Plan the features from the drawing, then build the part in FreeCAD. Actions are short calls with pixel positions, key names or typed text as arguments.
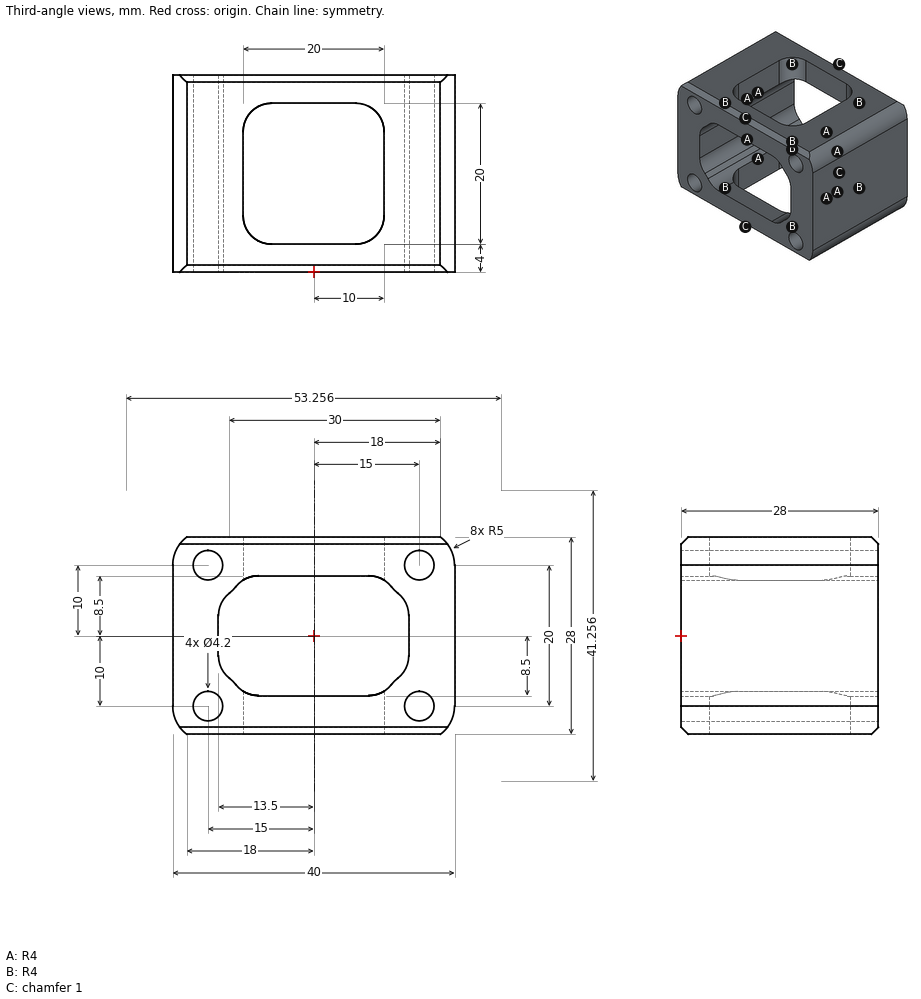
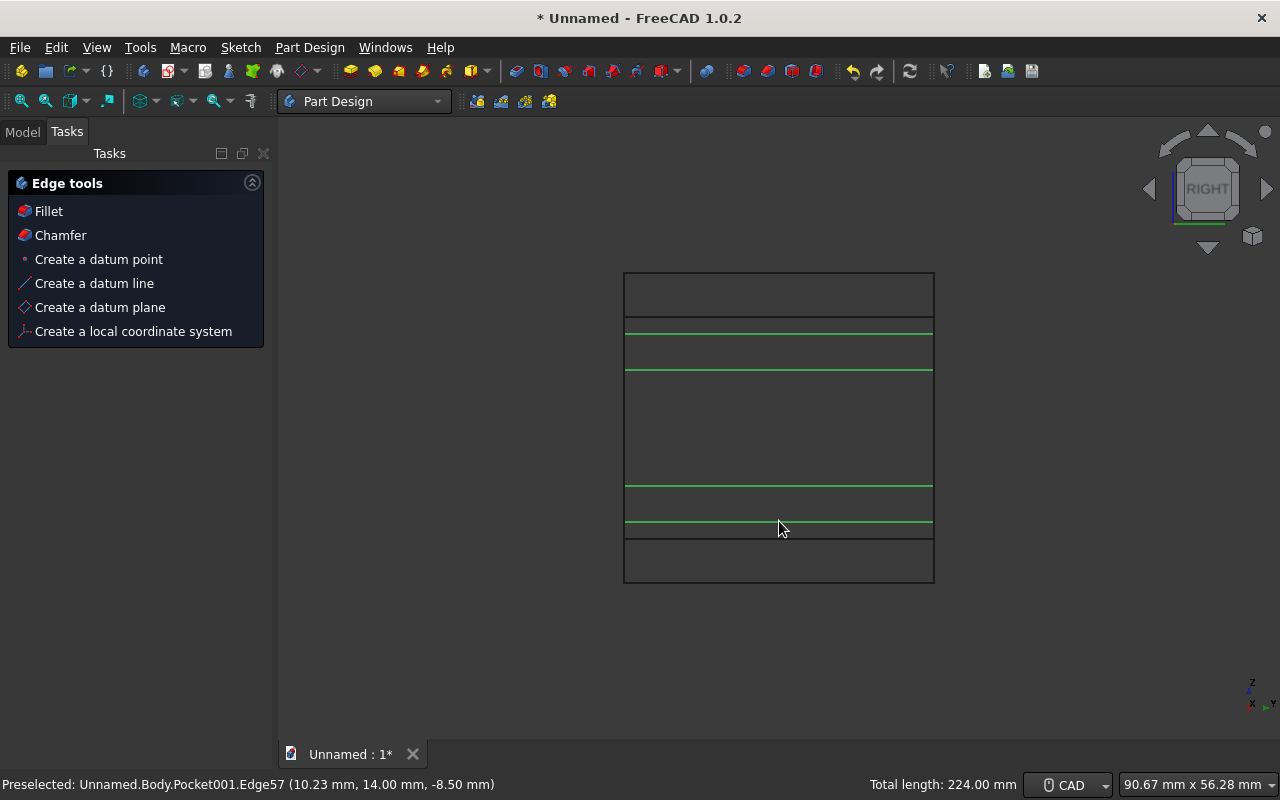
key(v)
key(1)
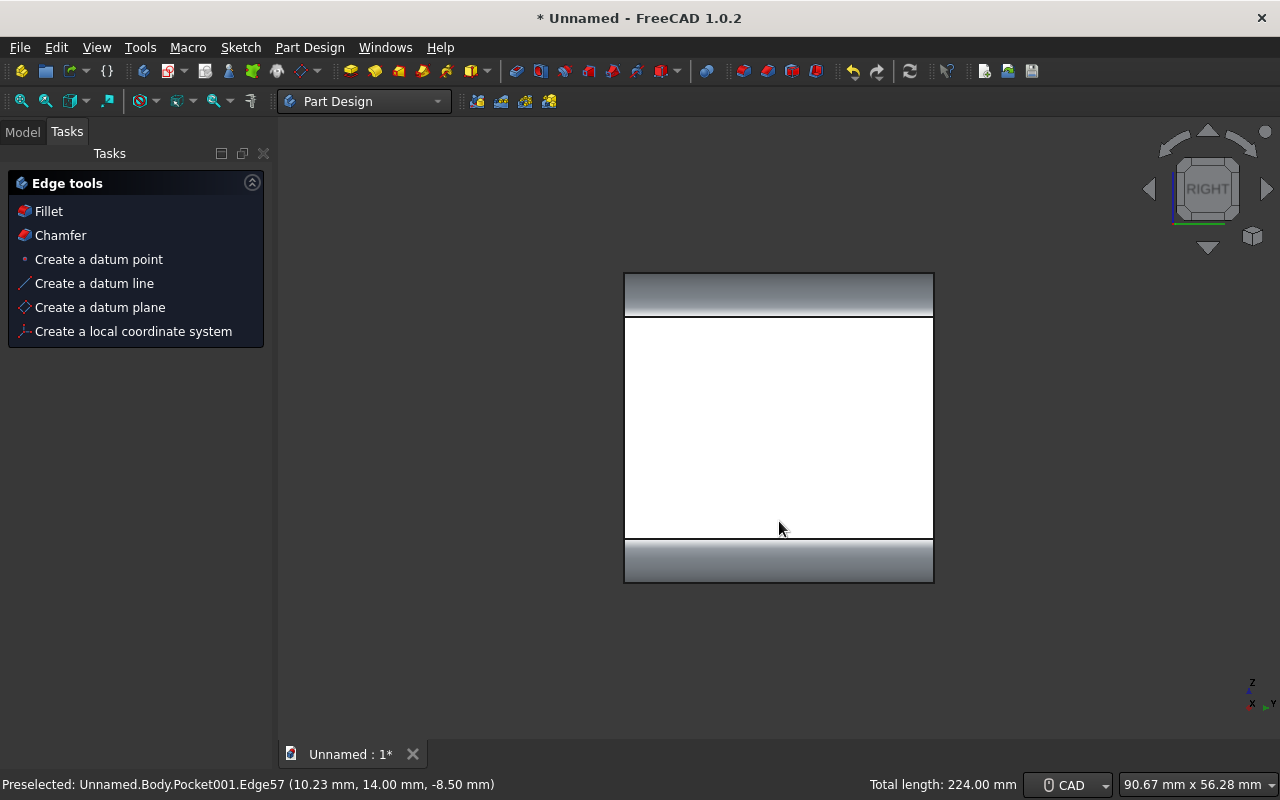
click(744, 72)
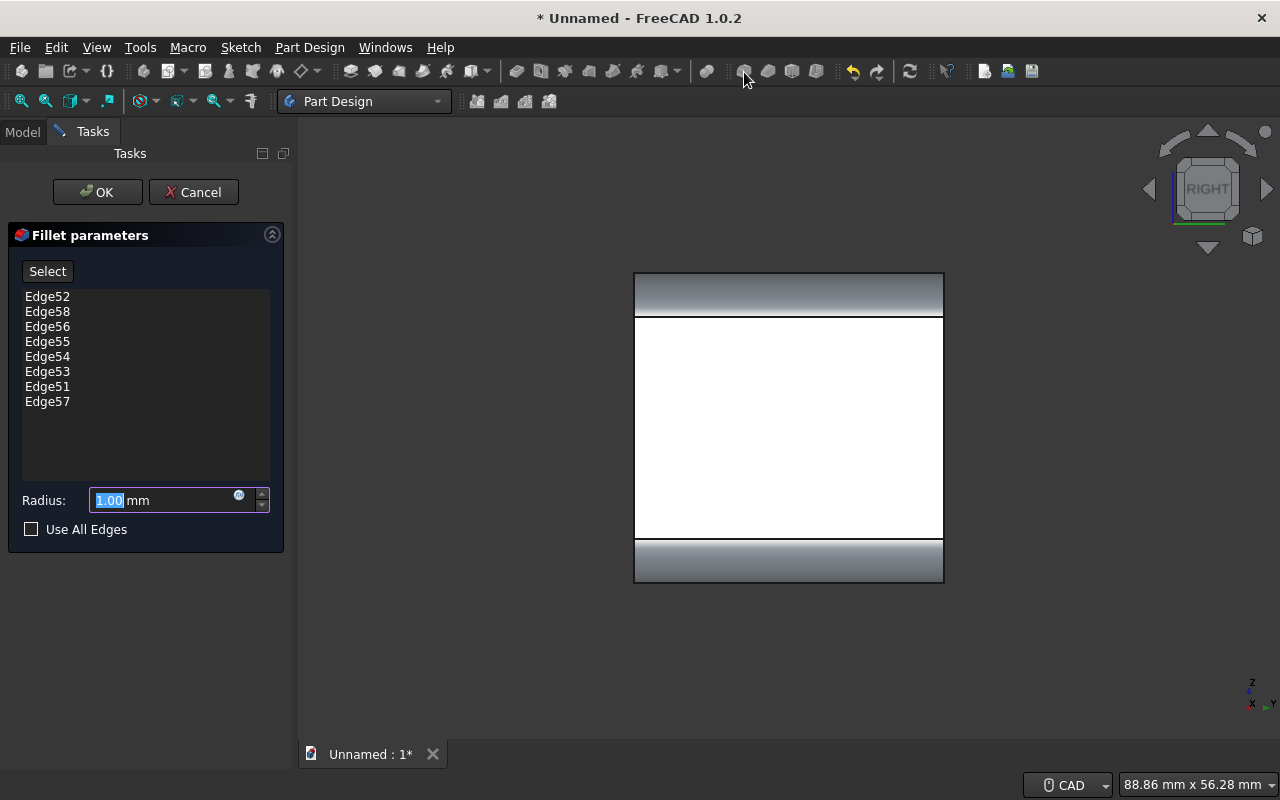
text(4)
key(Tab)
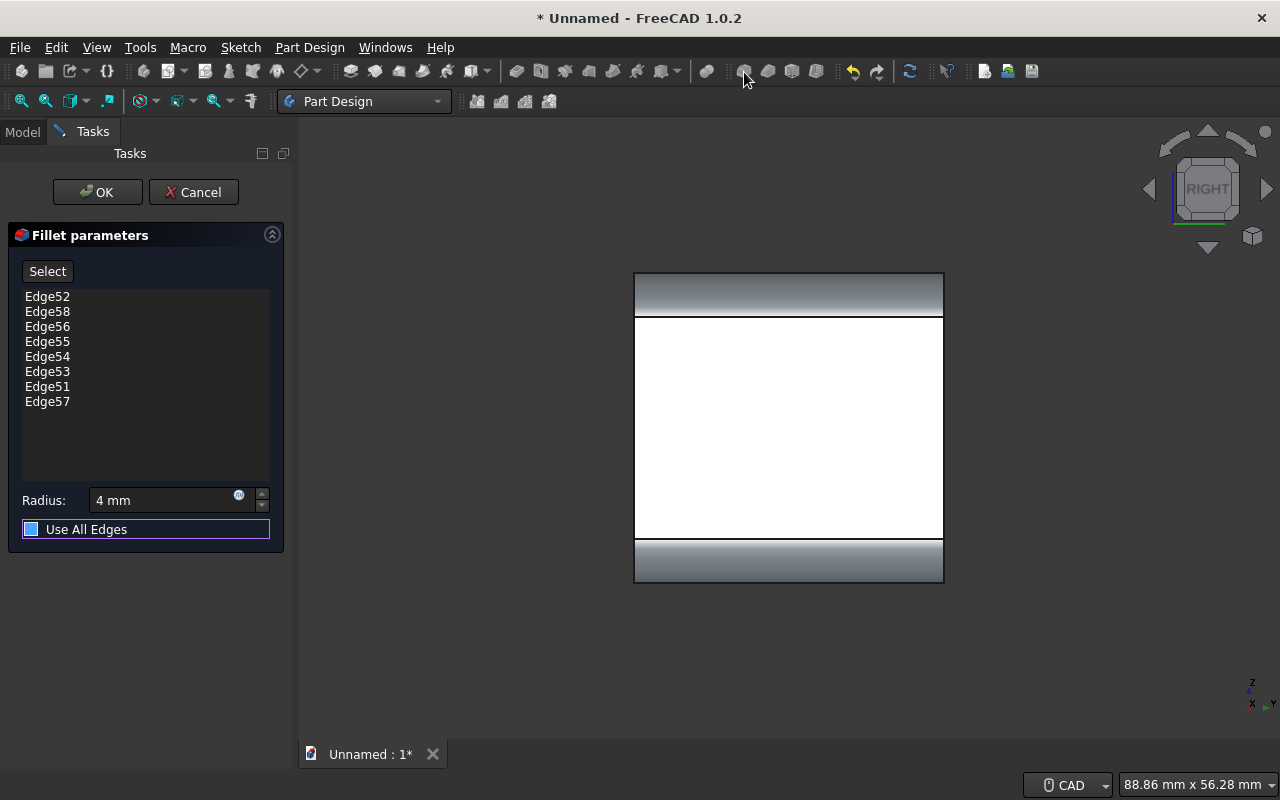
click(98, 192)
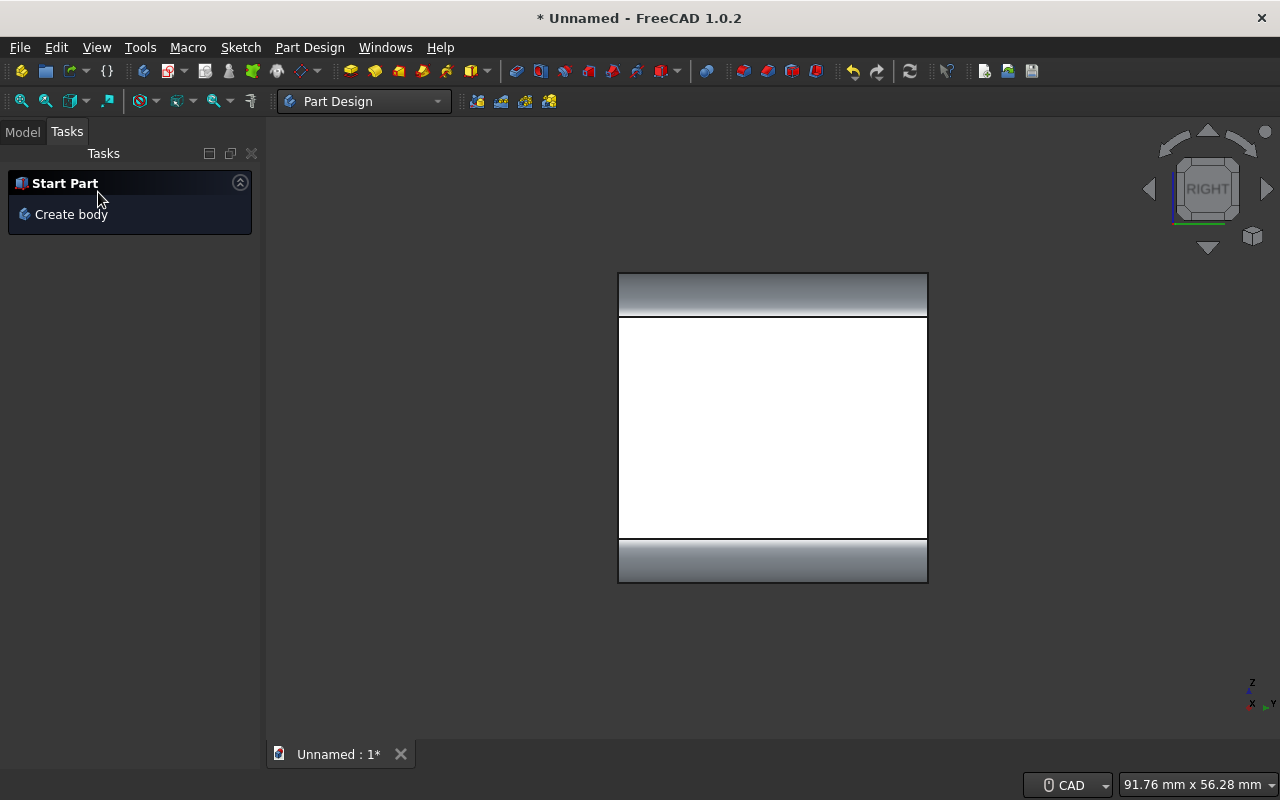
key(0)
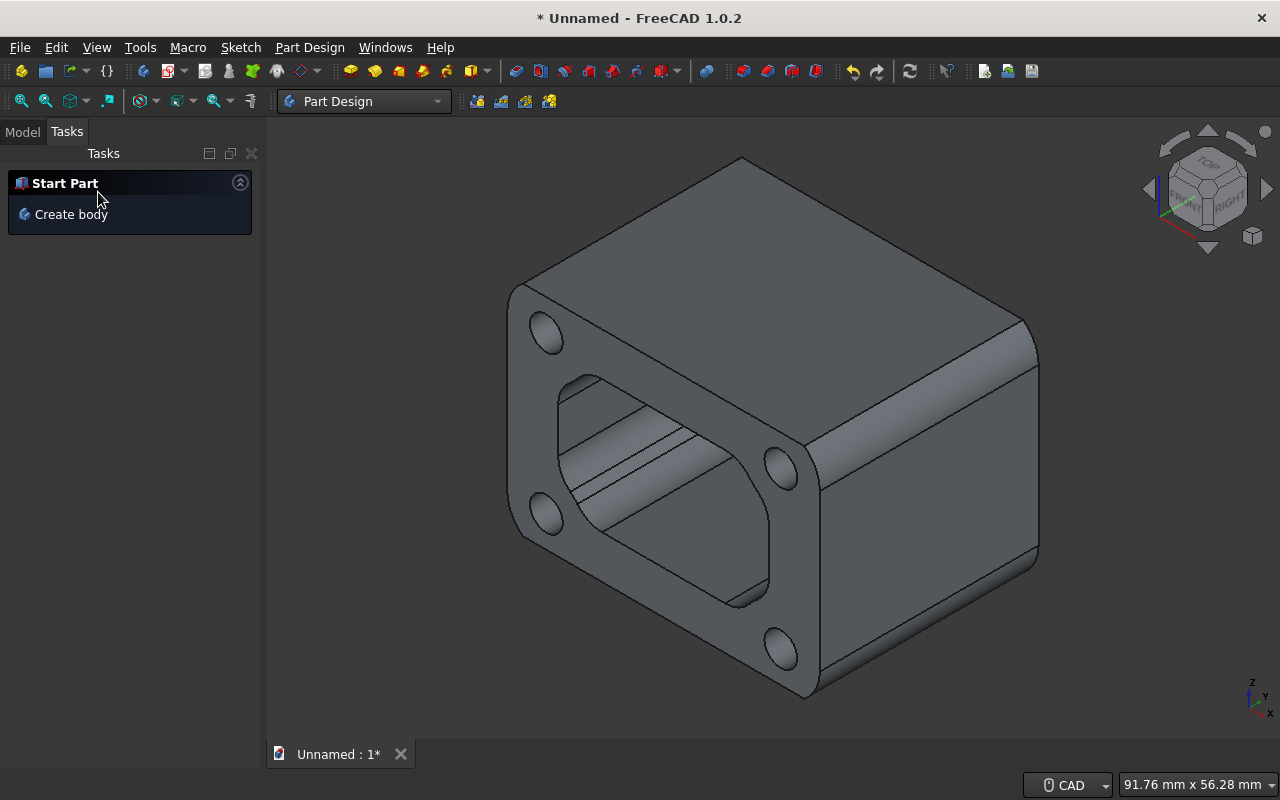
click(773, 301)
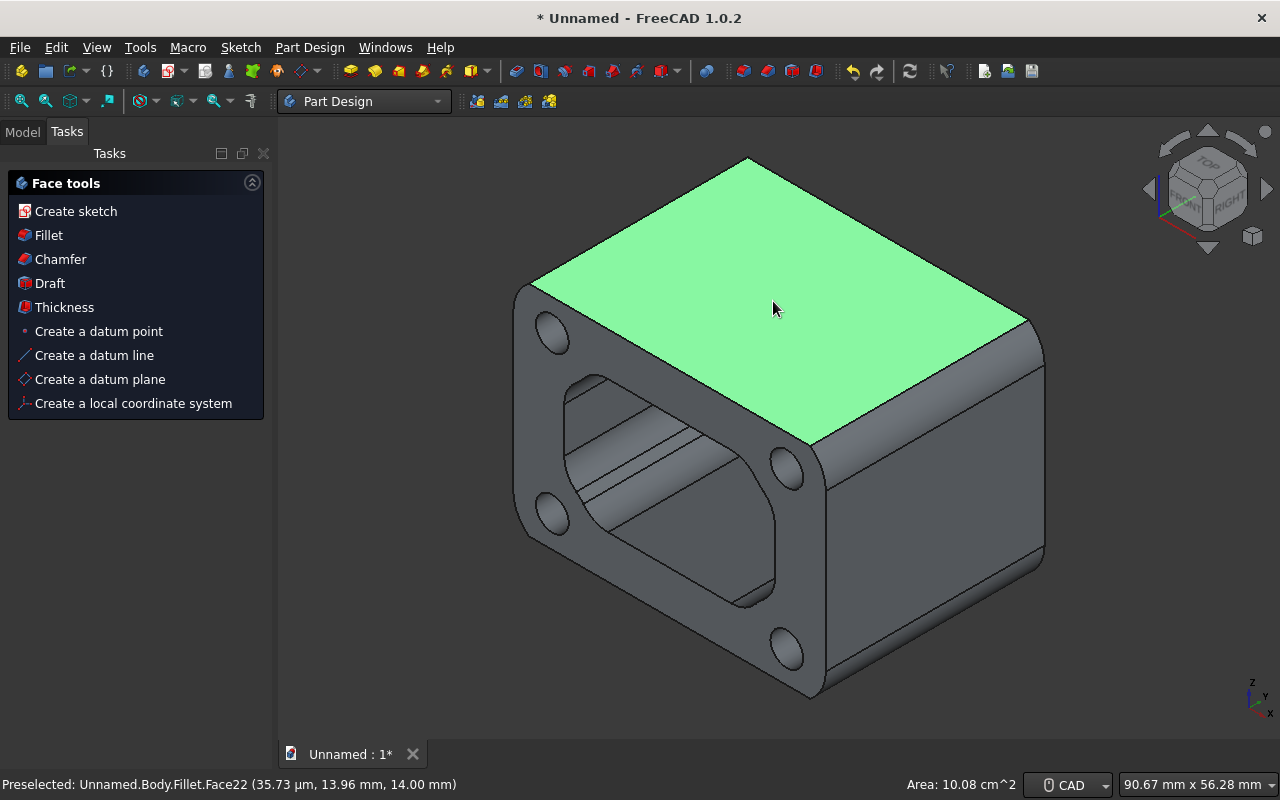
click(168, 72)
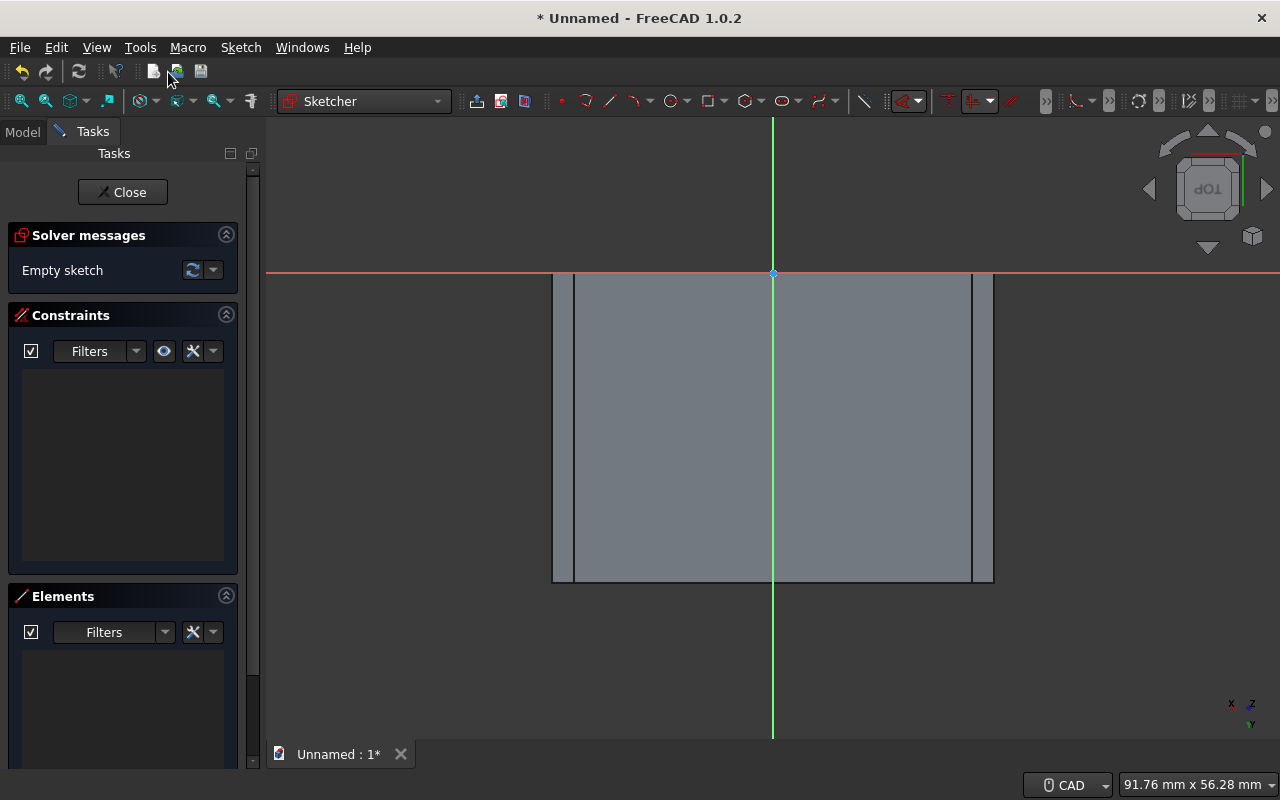
scroll(912, 361, up, 2)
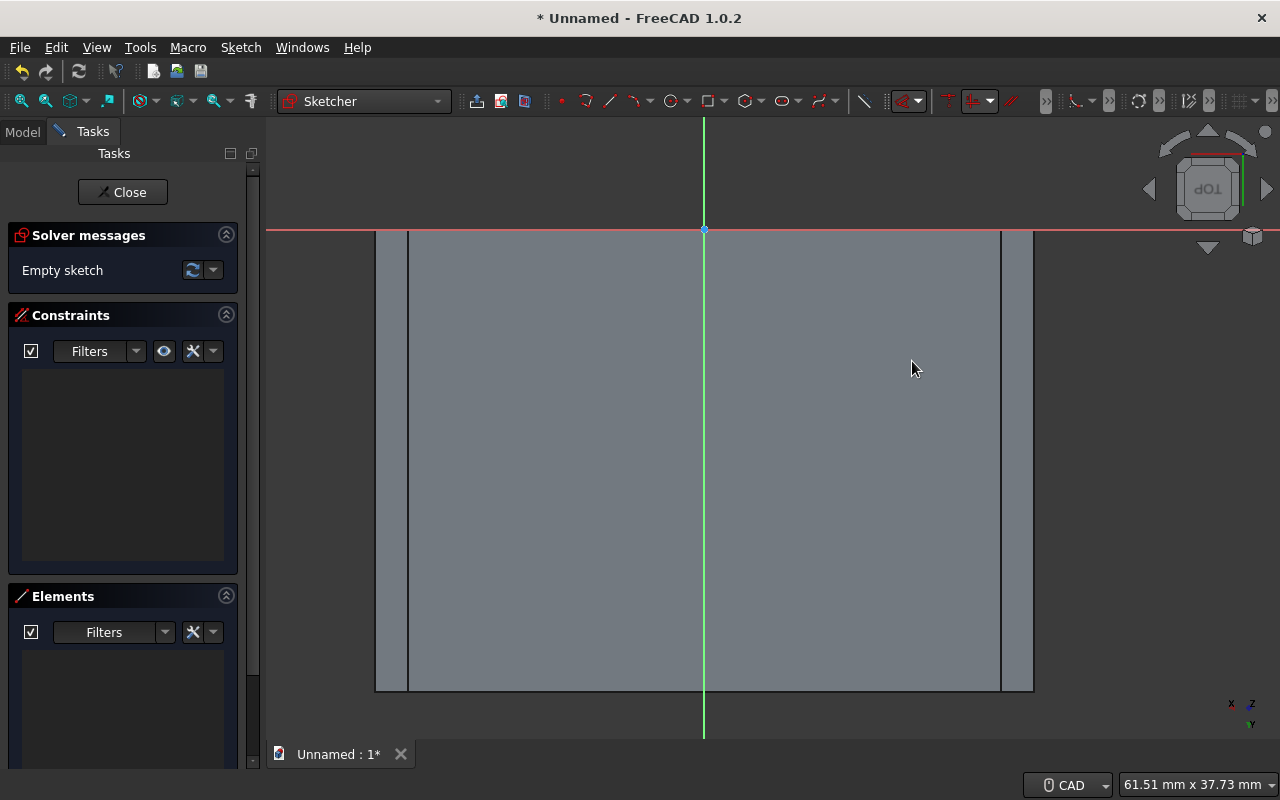
key(g)
key(r)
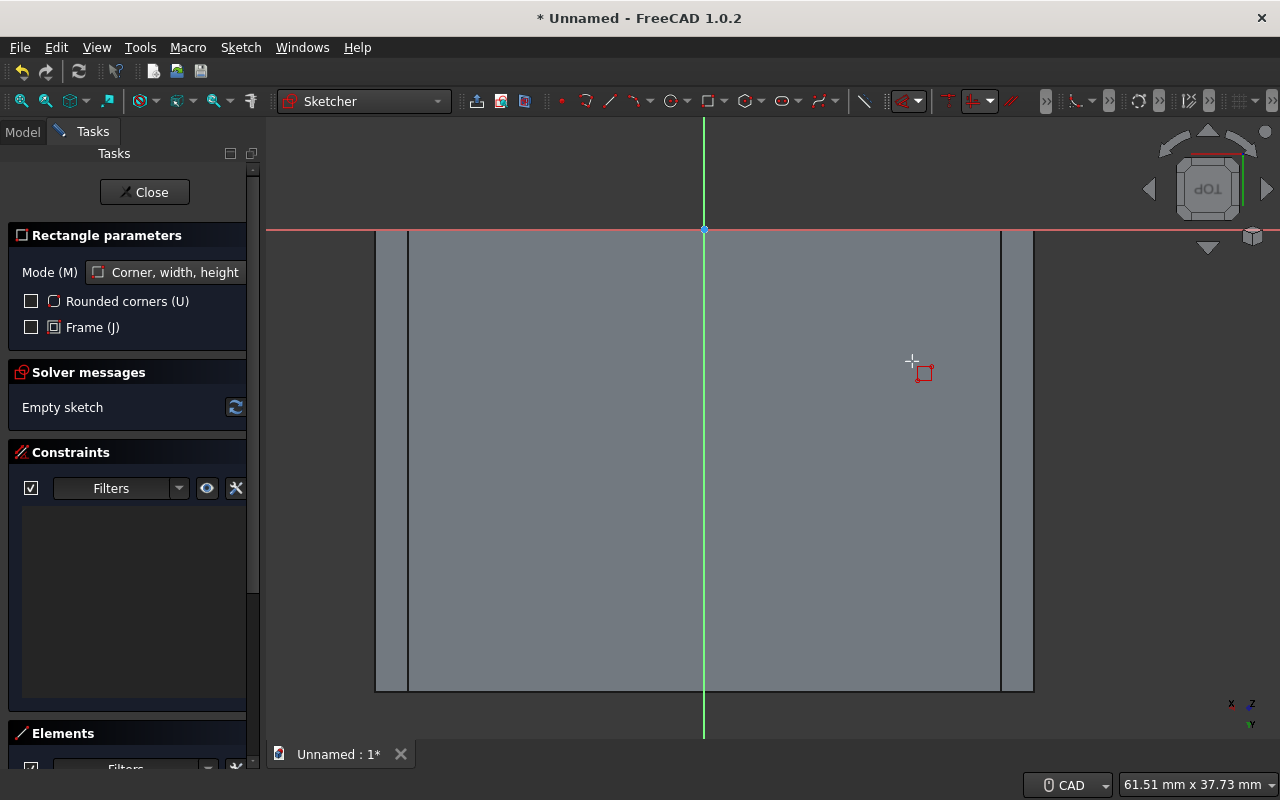
click(539, 296)
click(869, 626)
key(Escape)